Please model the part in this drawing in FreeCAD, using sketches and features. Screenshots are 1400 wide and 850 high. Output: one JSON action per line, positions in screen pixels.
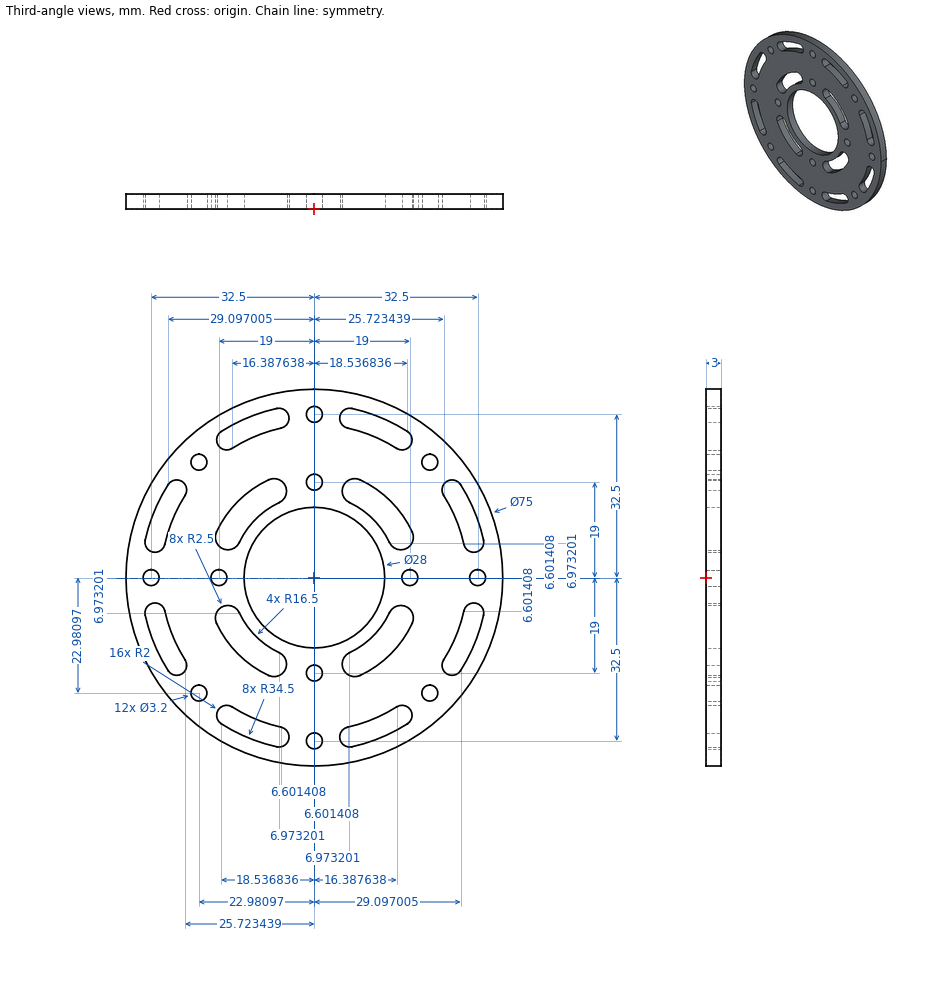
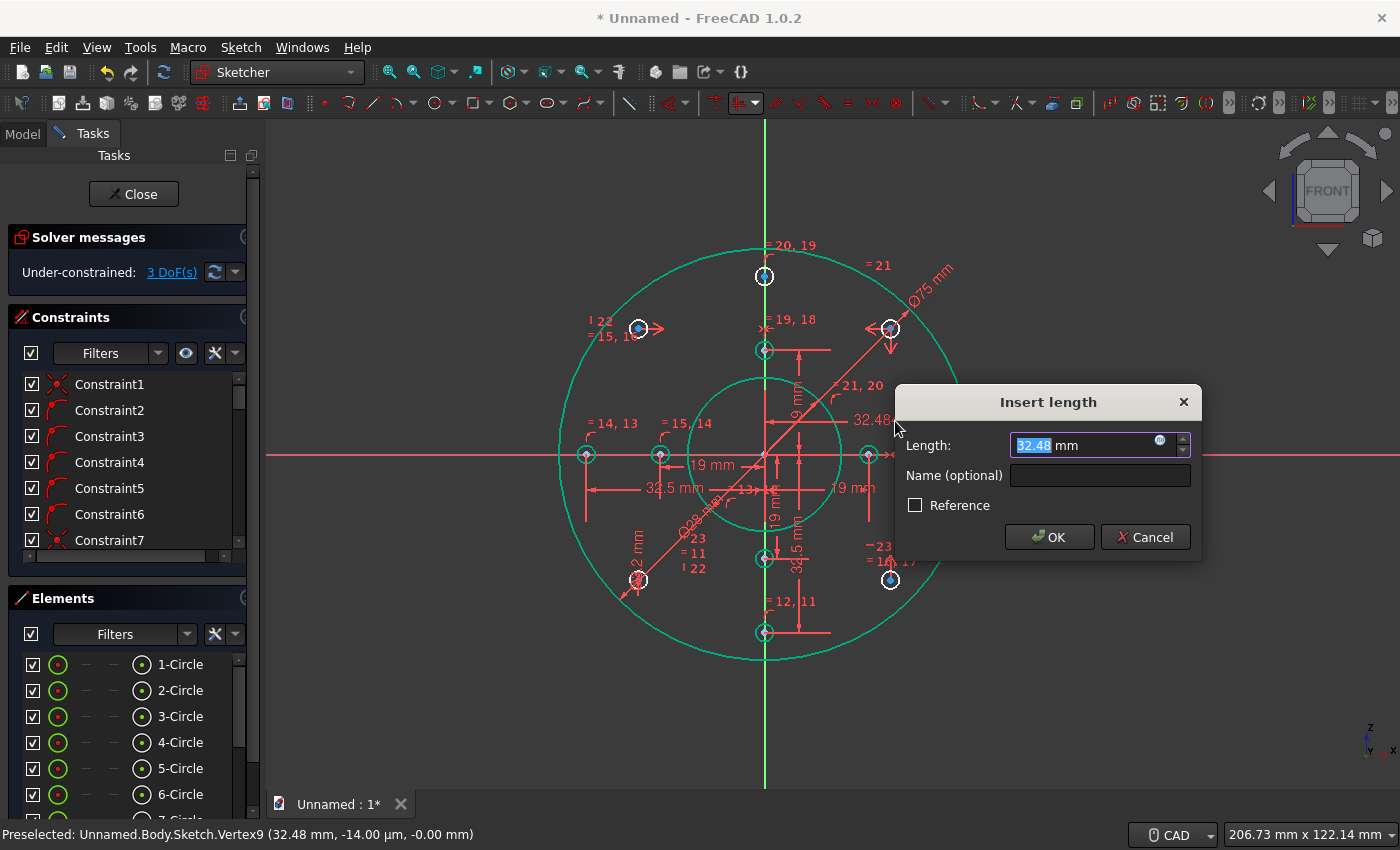
{"action": "type", "text": "32.5"}
{"action": "key", "text": "Return"}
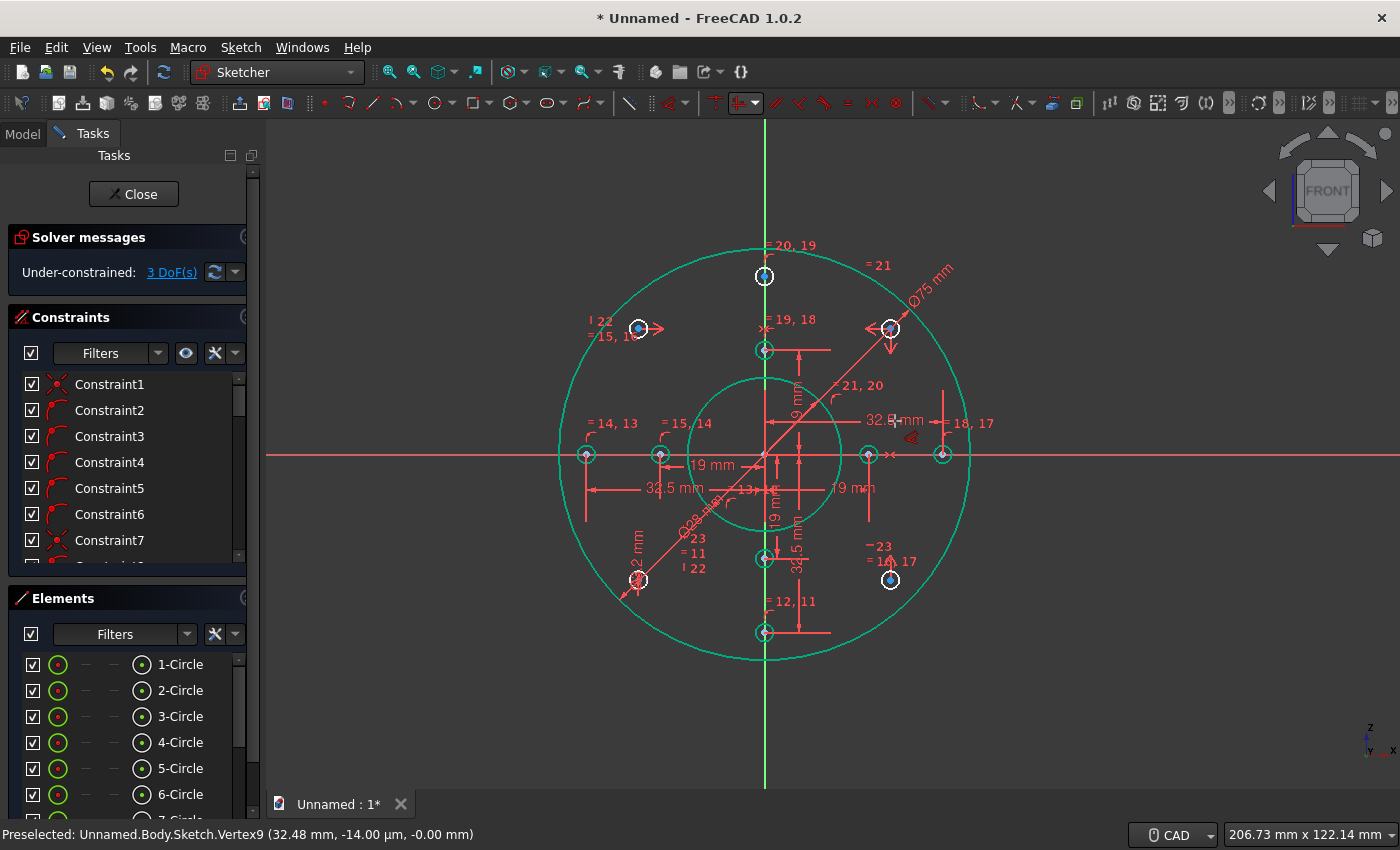
{"action": "left_click", "coordinate": [765, 277]}
{"action": "left_click", "coordinate": [799, 366]}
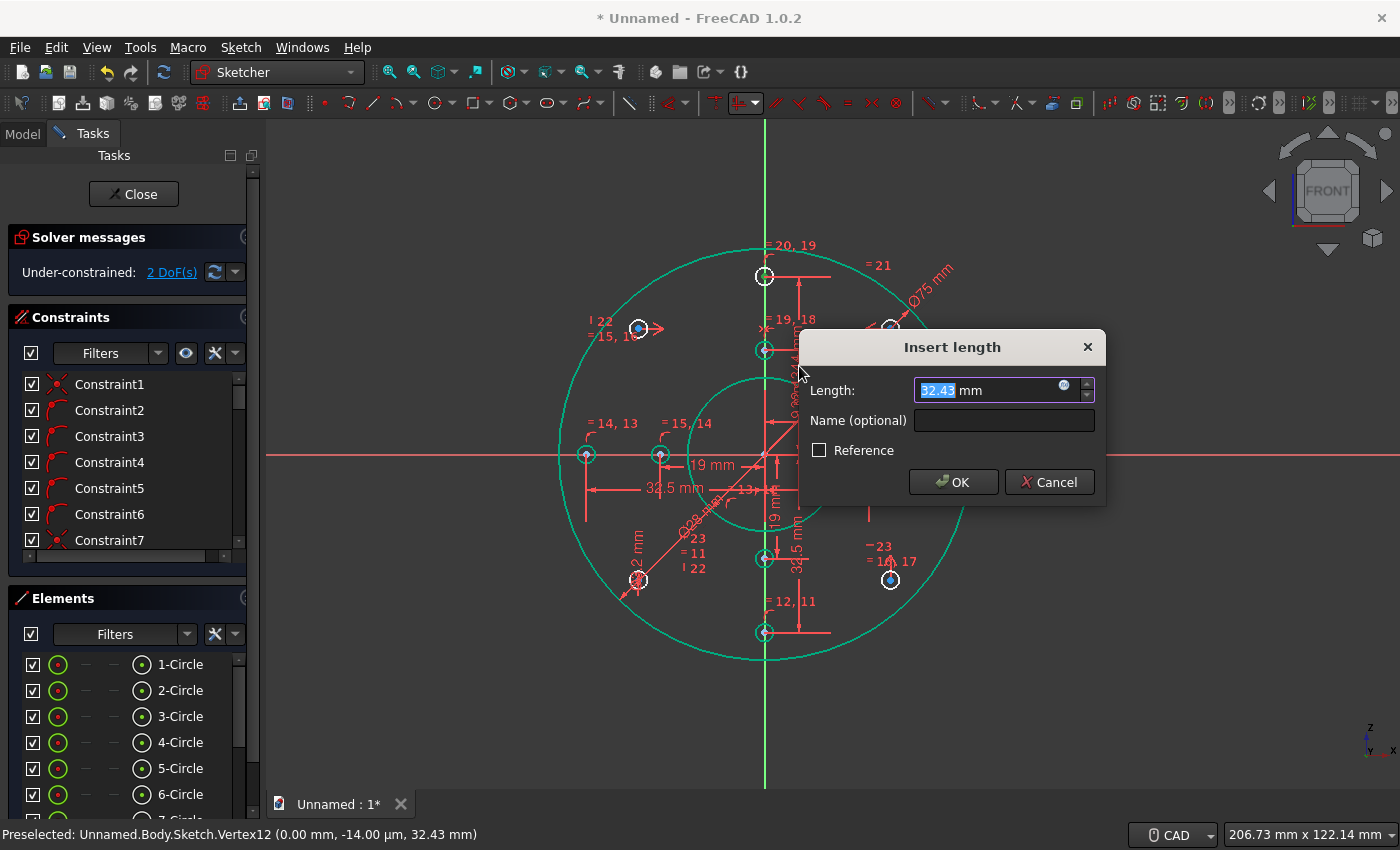
{"action": "type", "text": "32.5"}
{"action": "key", "text": "Return"}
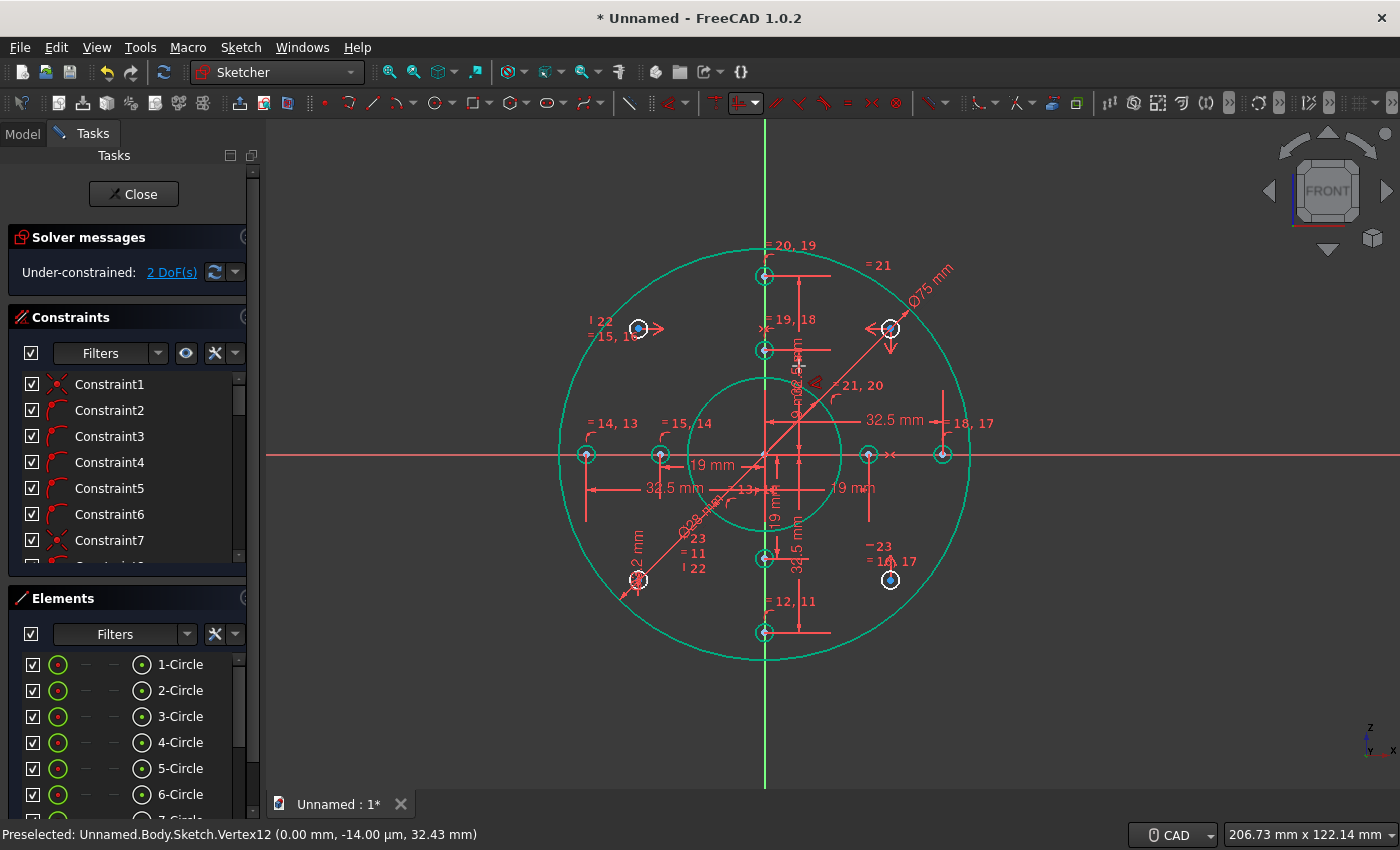
{"action": "left_click", "coordinate": [639, 580]}
{"action": "left_click", "coordinate": [702, 614]}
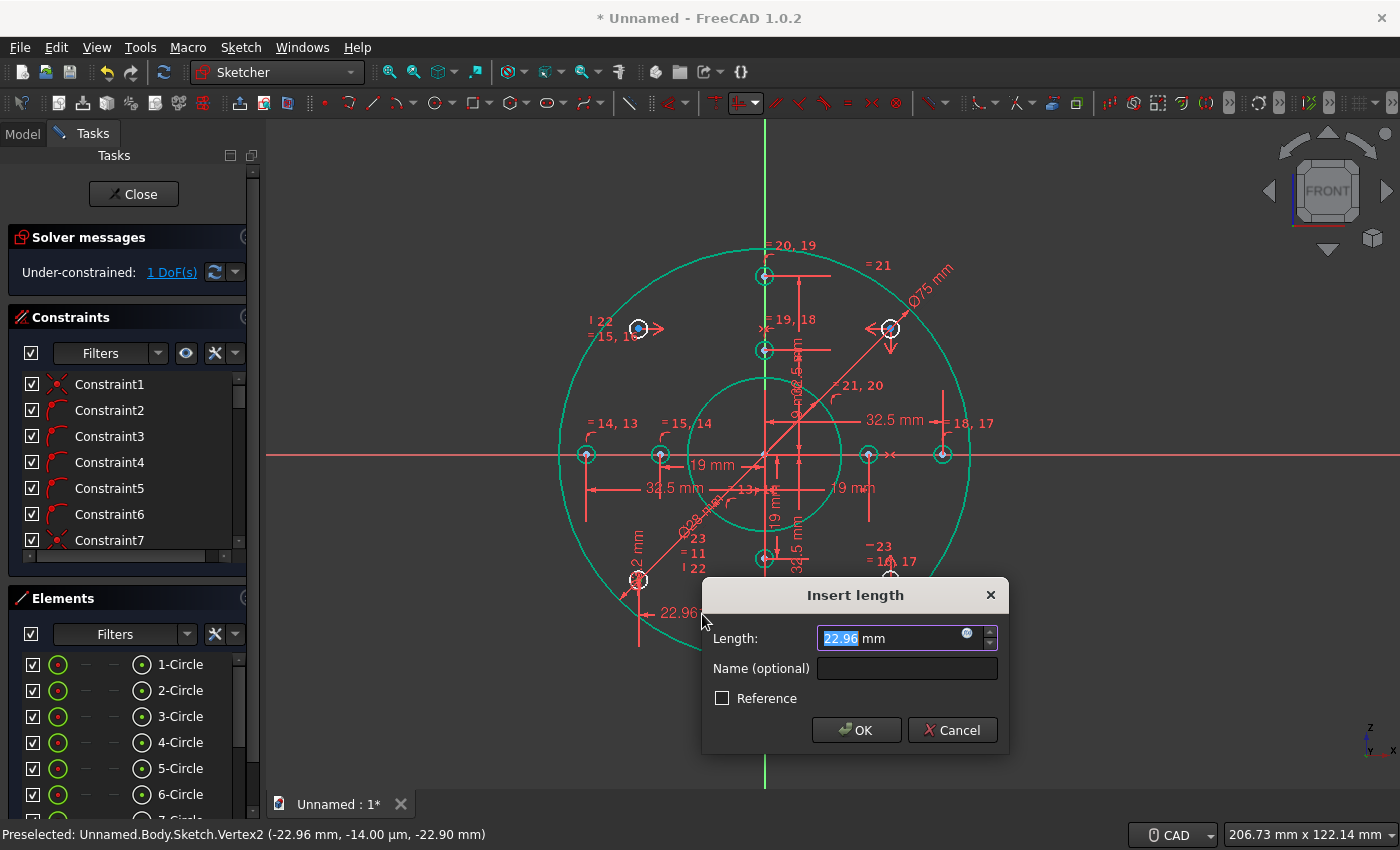
{"action": "type", "text": "22.98097"}
{"action": "key", "text": "Return"}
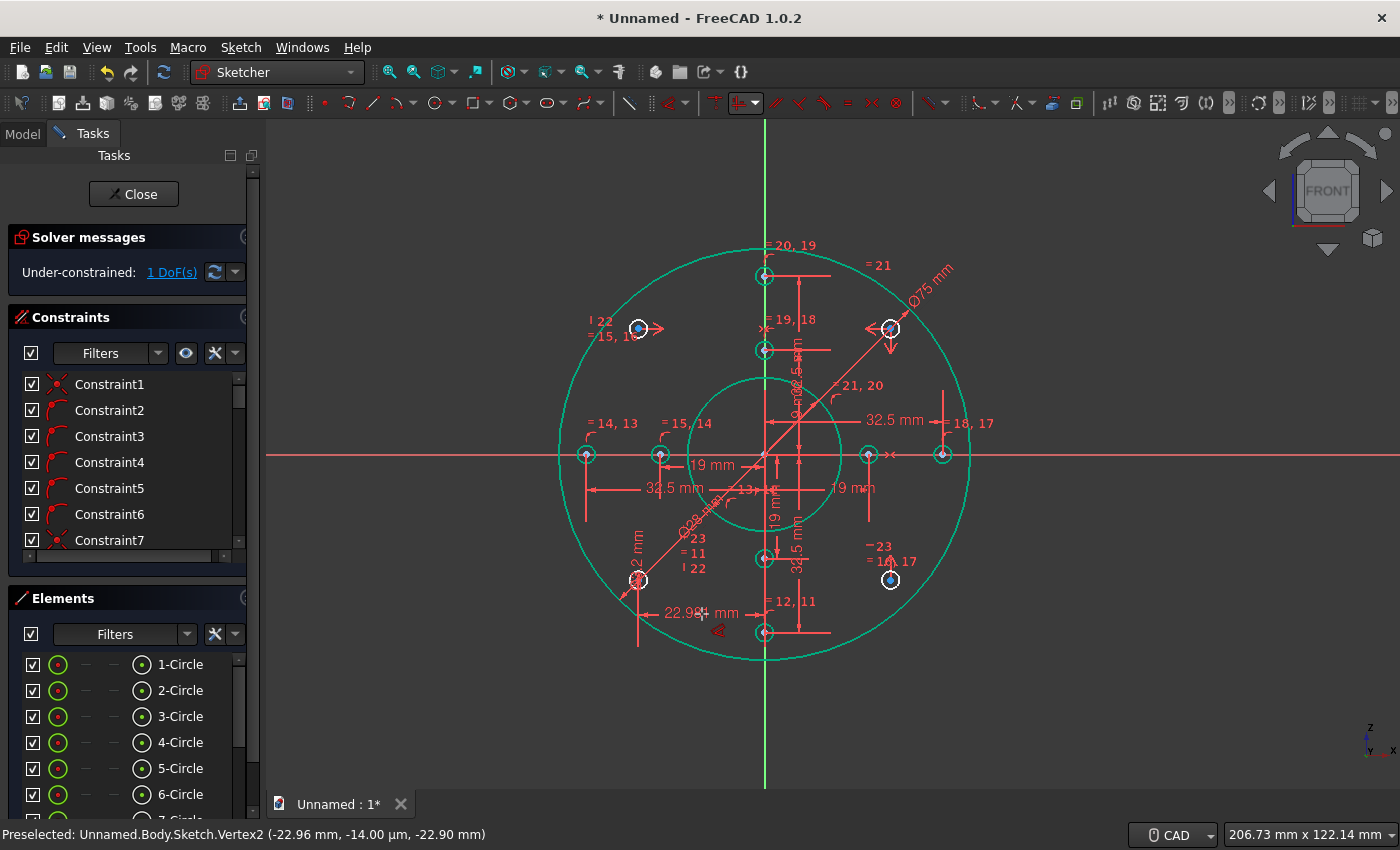
{"action": "left_click", "coordinate": [638, 580]}
{"action": "left_click", "coordinate": [604, 517]}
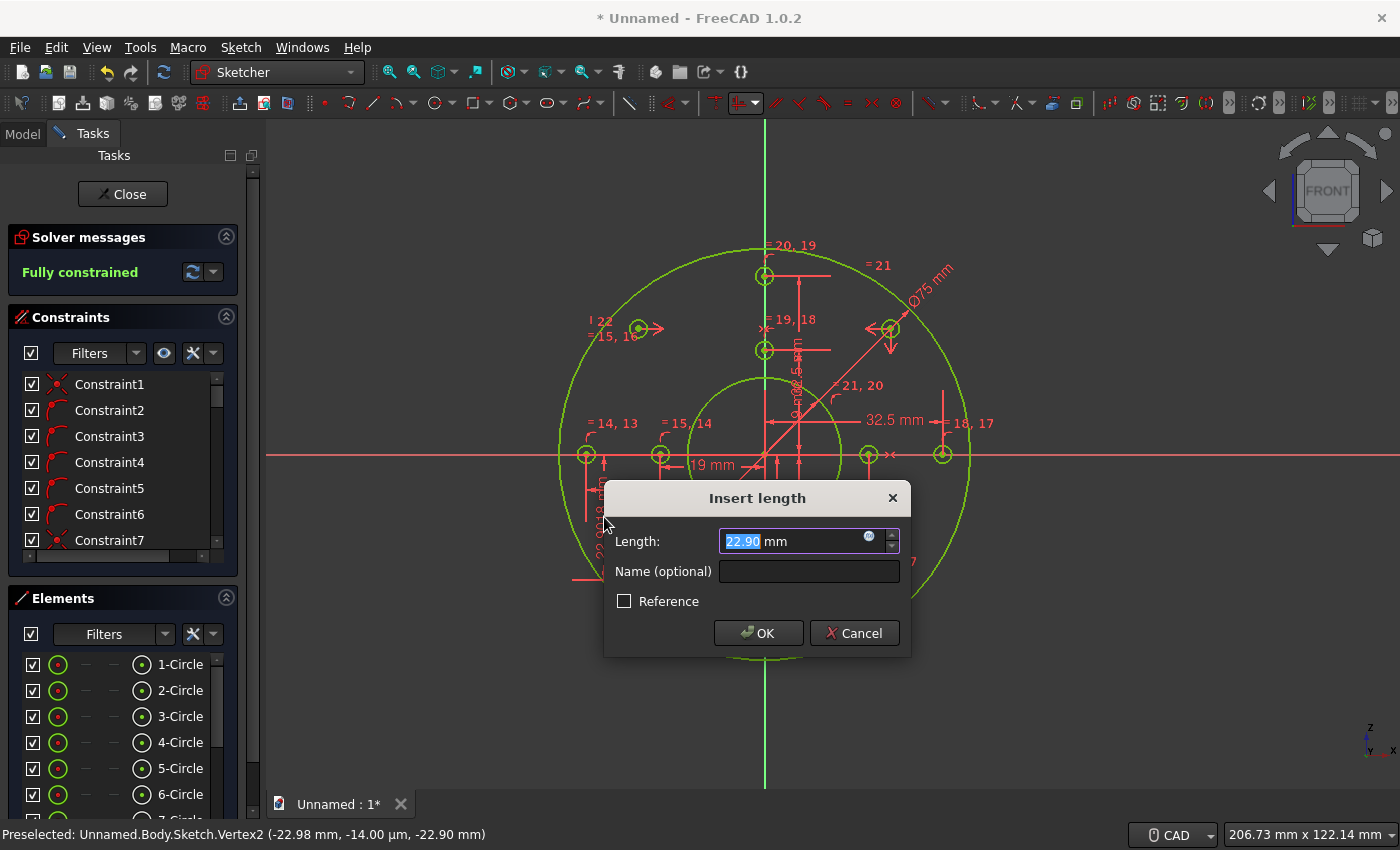
{"action": "type", "text": "22.98097"}
{"action": "key", "text": "Return"}
{"action": "key", "text": "Escape"}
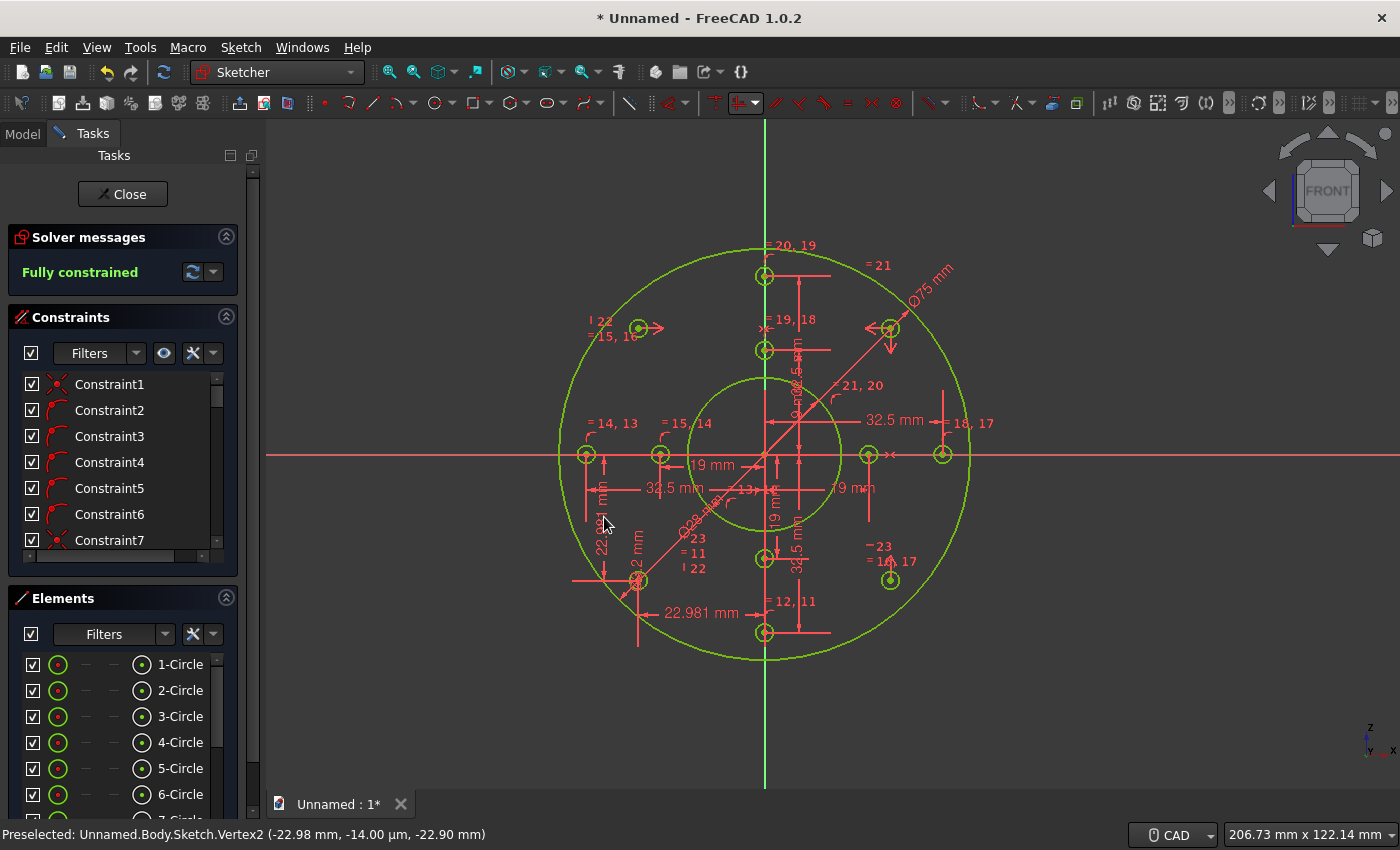
{"action": "left_click", "coordinate": [123, 194]}